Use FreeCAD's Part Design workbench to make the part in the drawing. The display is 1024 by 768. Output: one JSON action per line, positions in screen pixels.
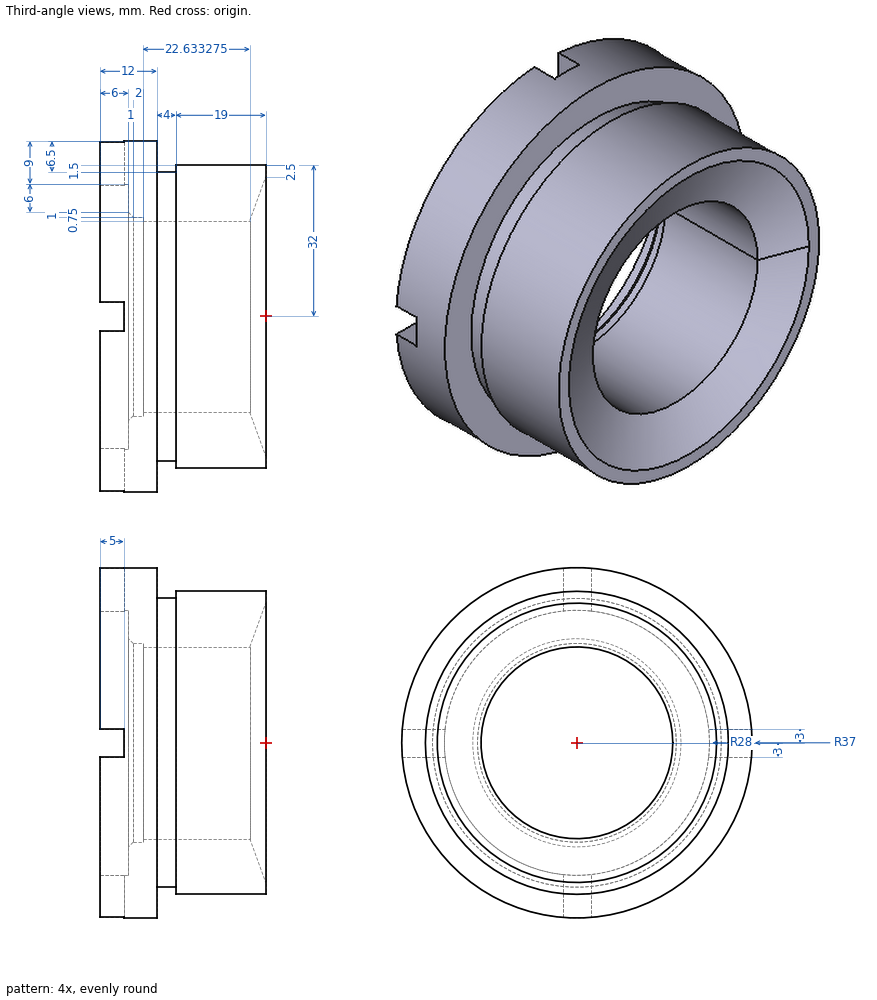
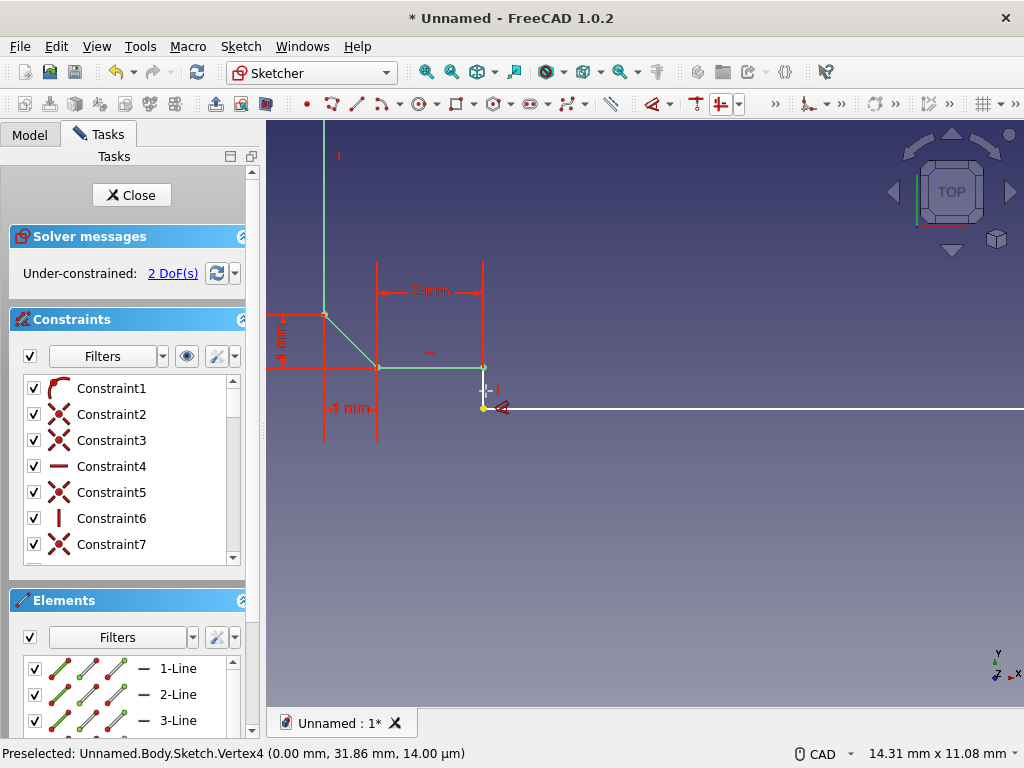
{"action": "left_click", "coordinate": [483, 388]}
{"action": "left_click", "coordinate": [449, 388]}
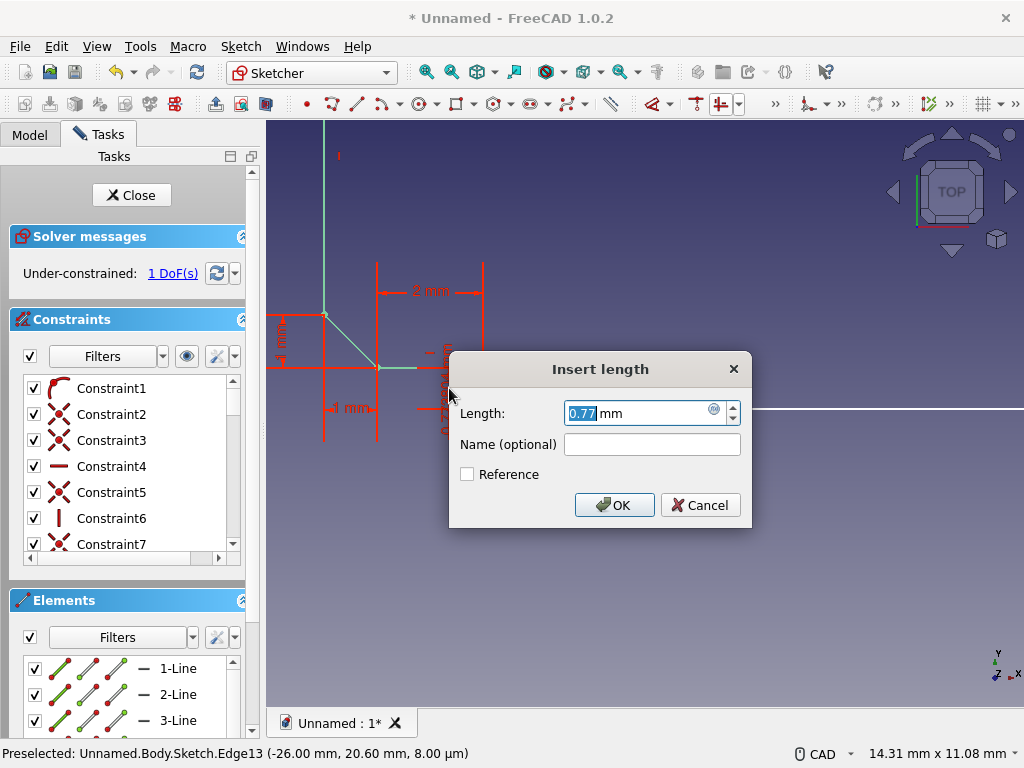
{"action": "type", "text": "0.75"}
{"action": "key", "text": "Return"}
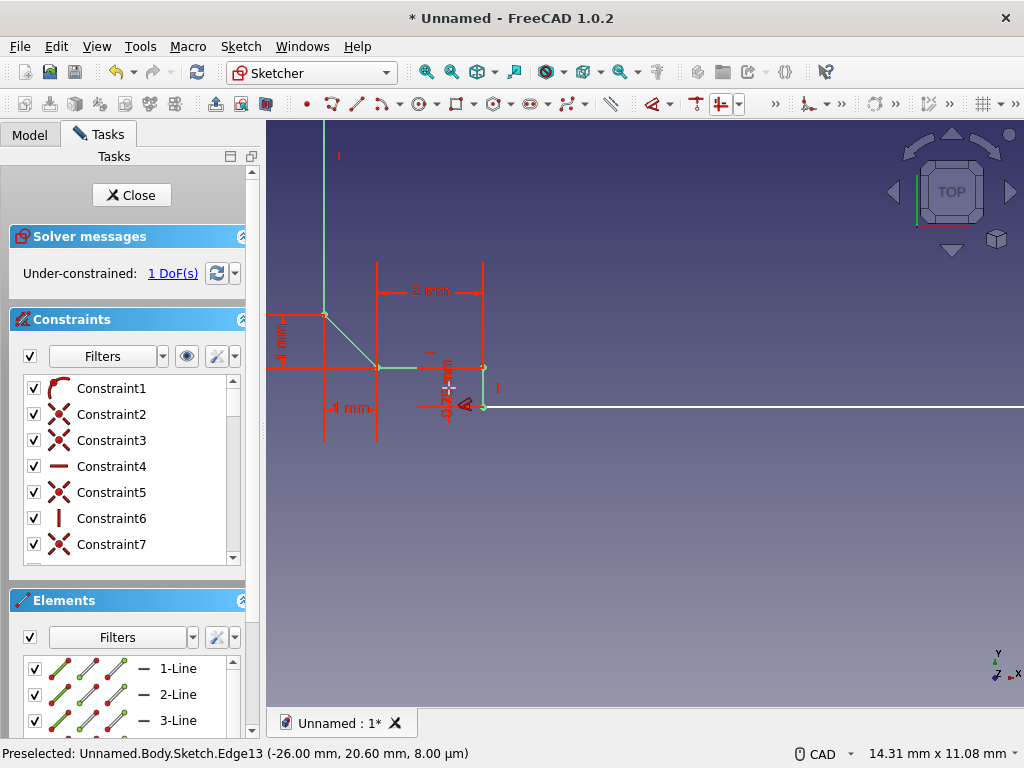
{"action": "scroll", "coordinate": [486, 392], "scroll_direction": "down", "scroll_amount": 8}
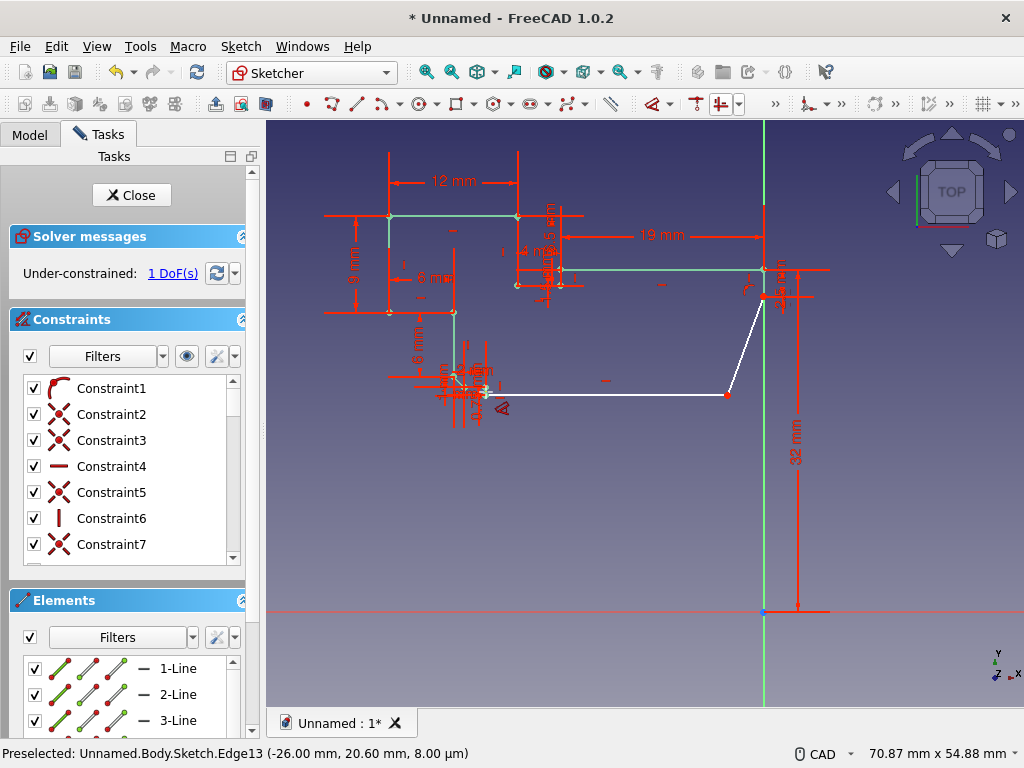
{"action": "left_click", "coordinate": [558, 395]}
{"action": "left_click", "coordinate": [607, 361]}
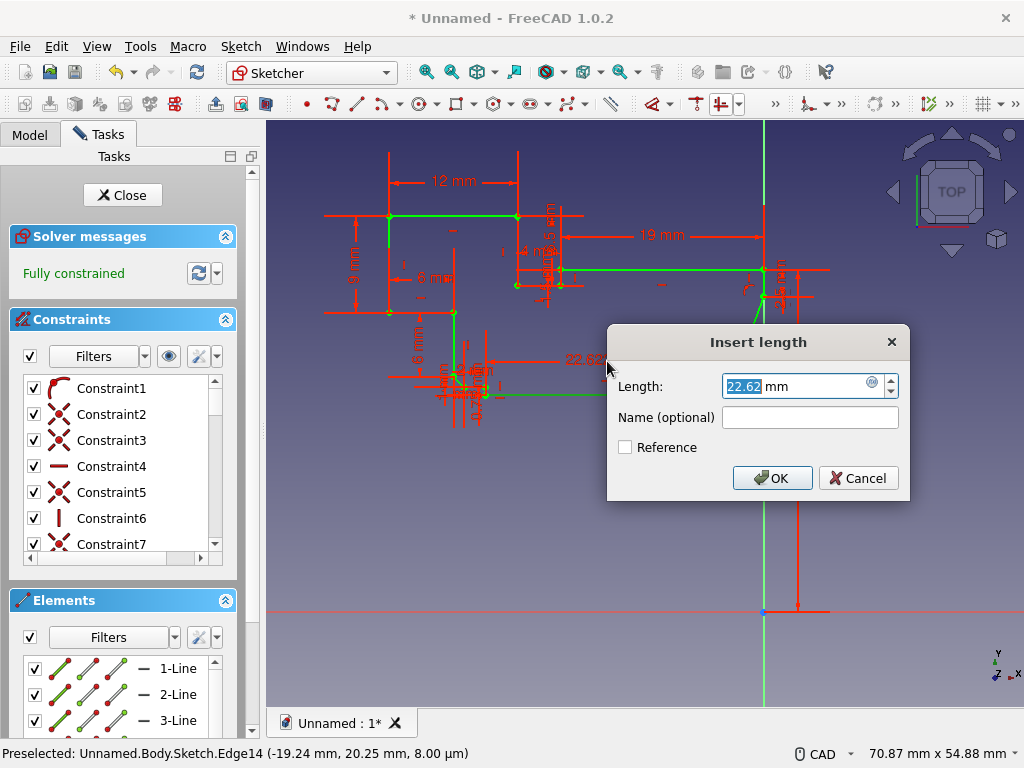
{"action": "type", "text": "22.633275"}
{"action": "key", "text": "Return"}
{"action": "key", "text": "Escape"}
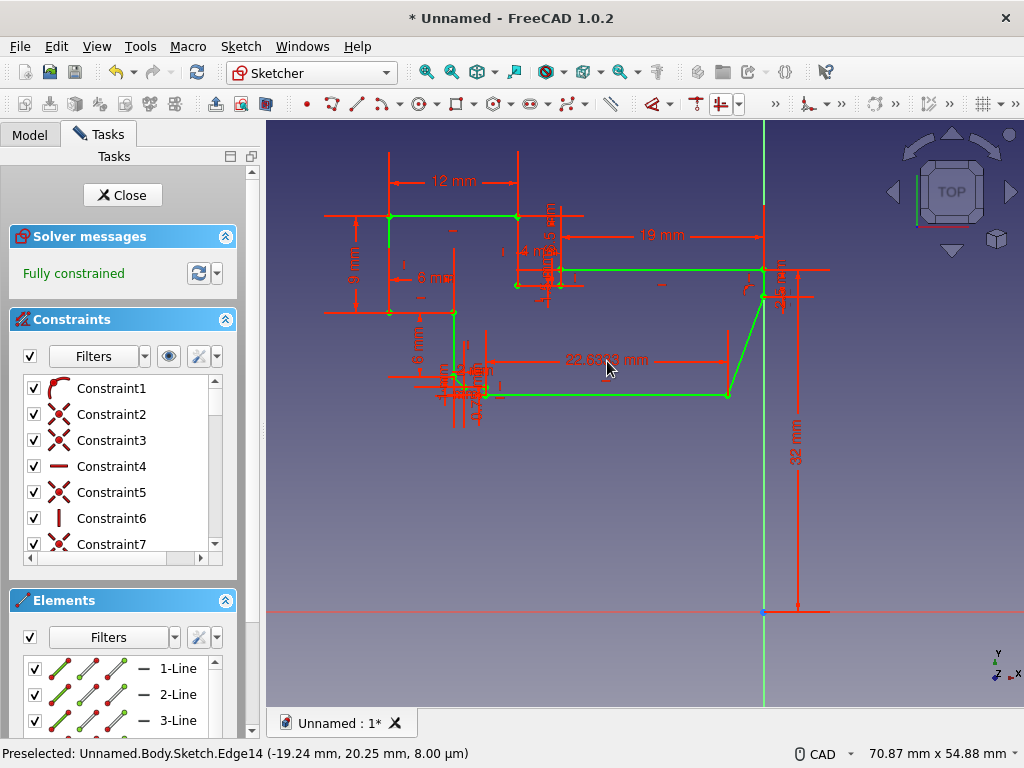
{"action": "left_click", "coordinate": [123, 195]}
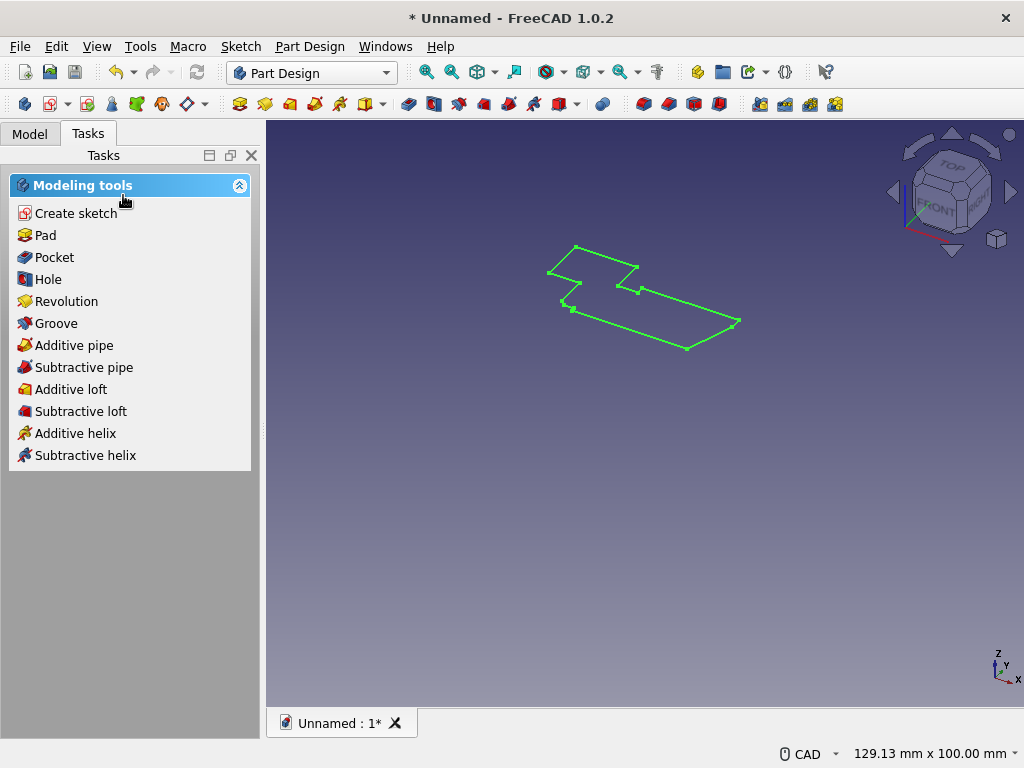
{"action": "left_click", "coordinate": [265, 104]}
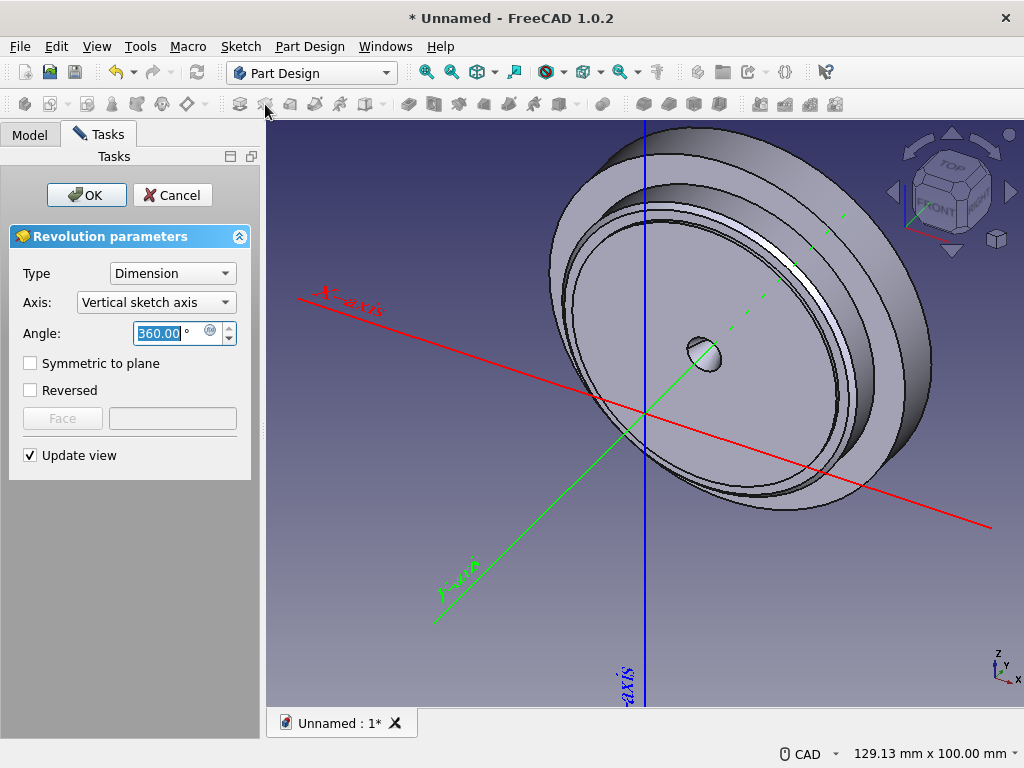
{"action": "left_click", "coordinate": [157, 302]}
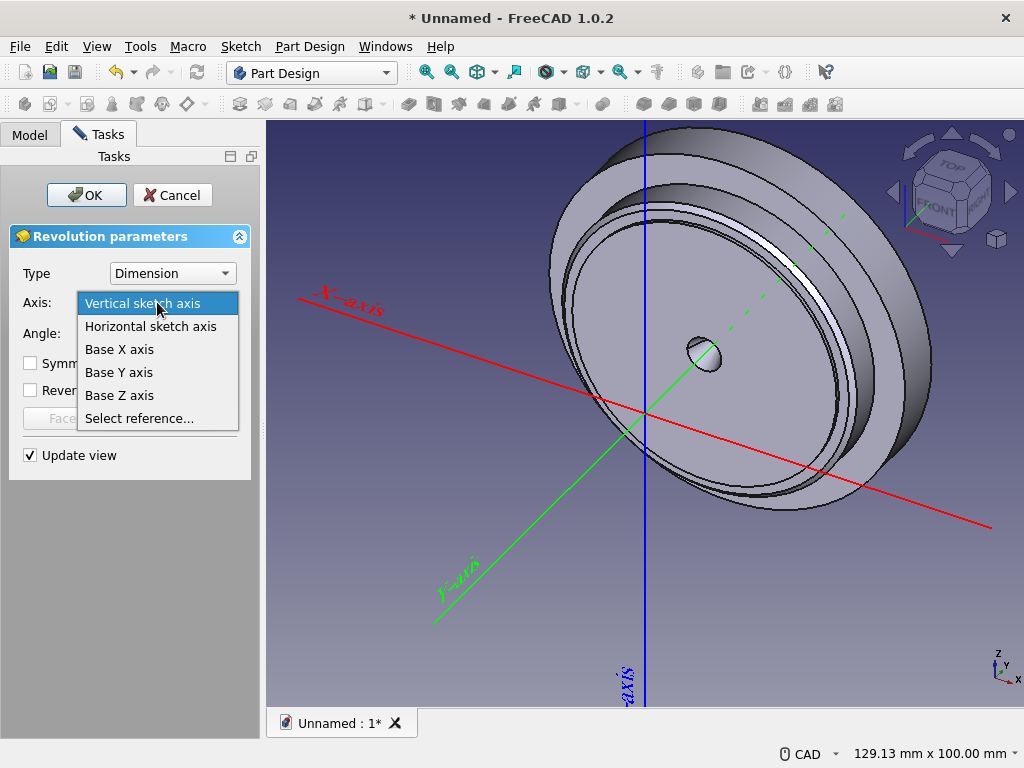
{"action": "left_click", "coordinate": [156, 326]}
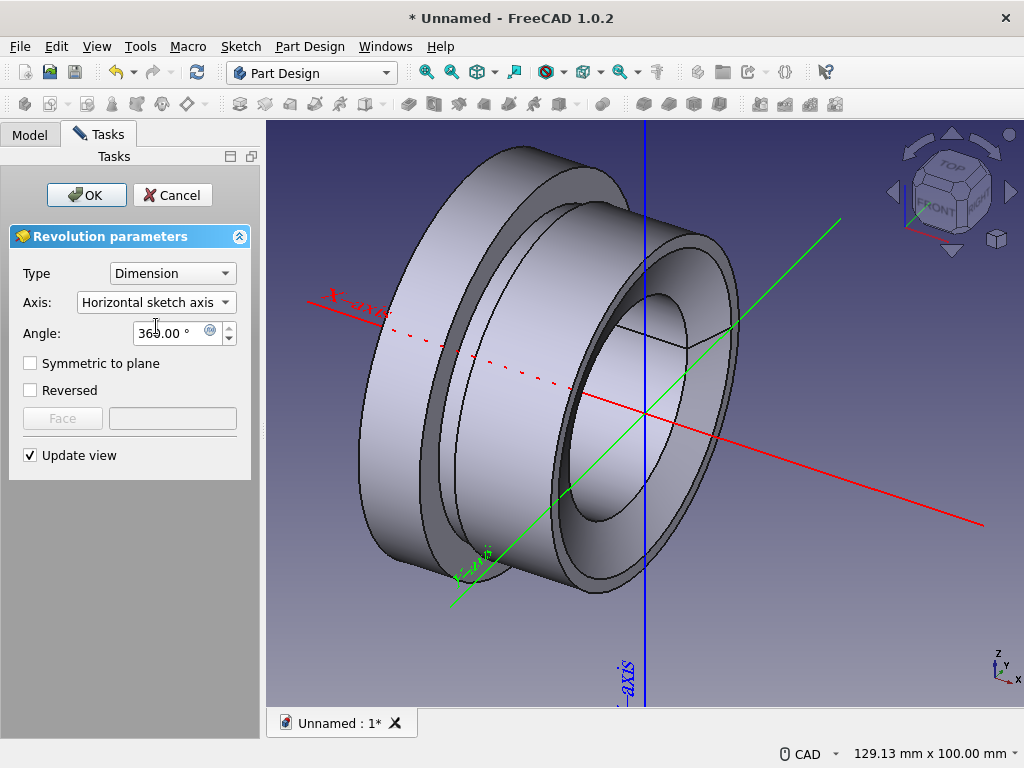
{"action": "left_click", "coordinate": [87, 195]}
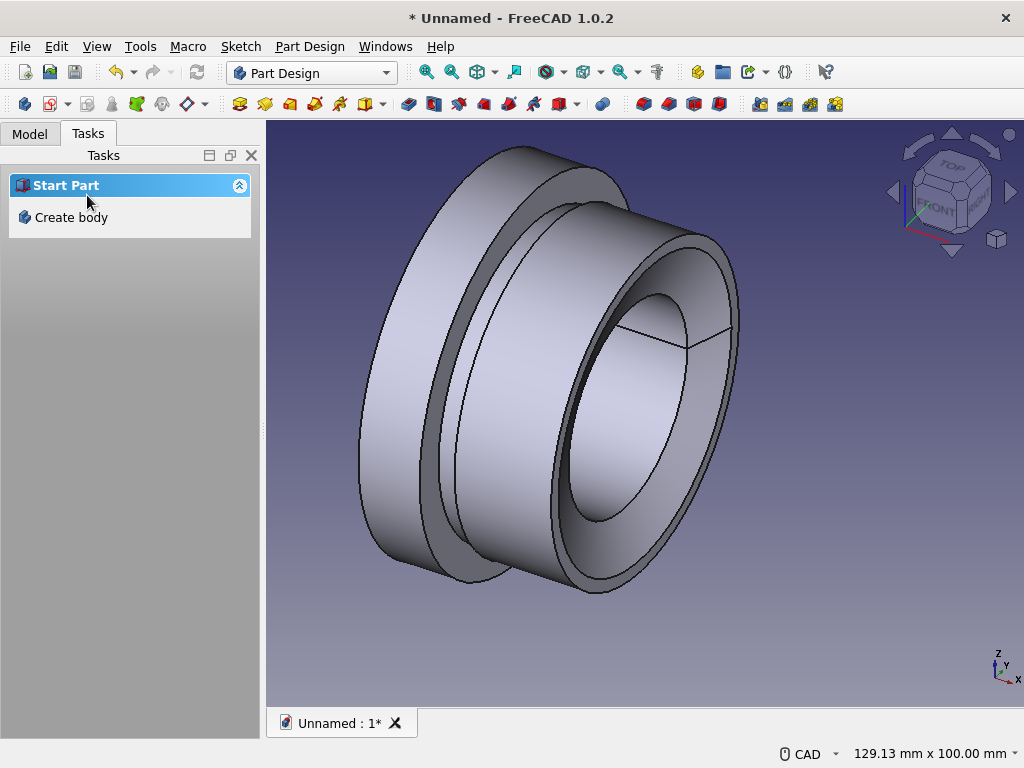
{"action": "left_click", "coordinate": [427, 72]}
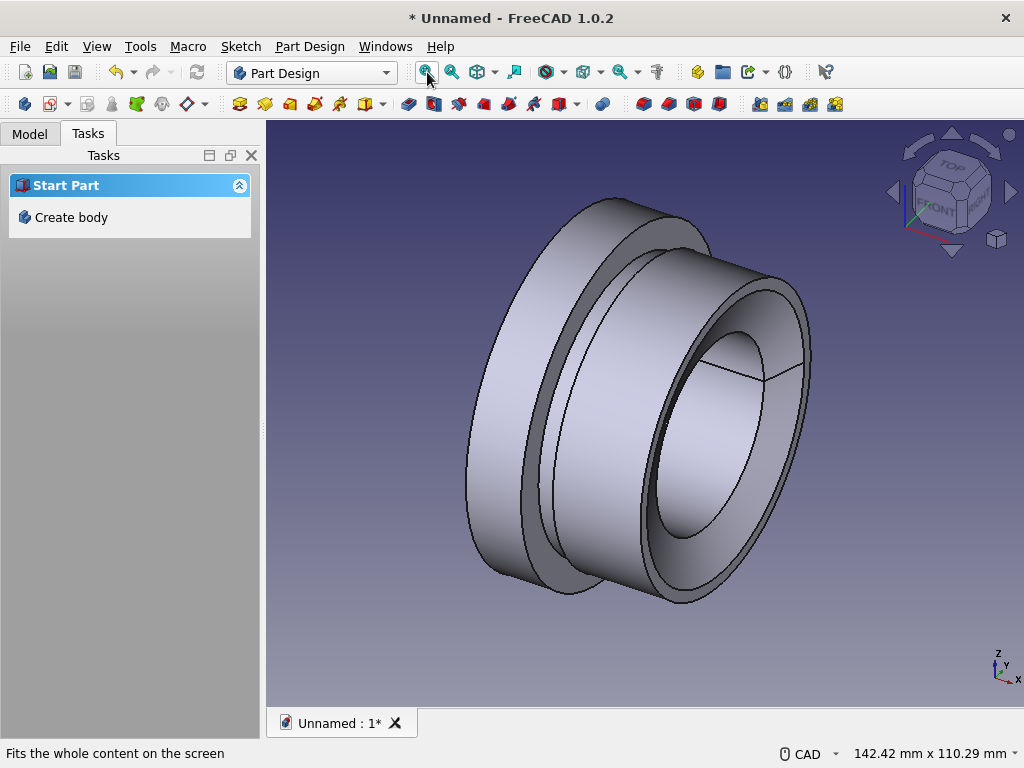
{"action": "key", "text": "6"}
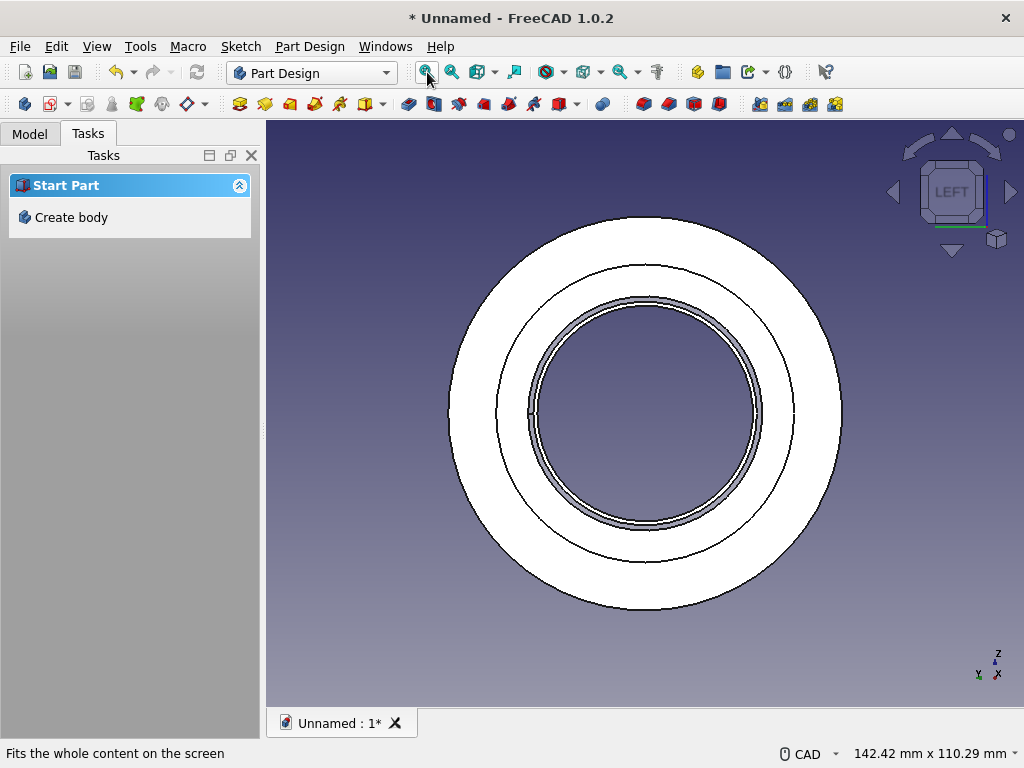
{"action": "left_click", "coordinate": [645, 581]}